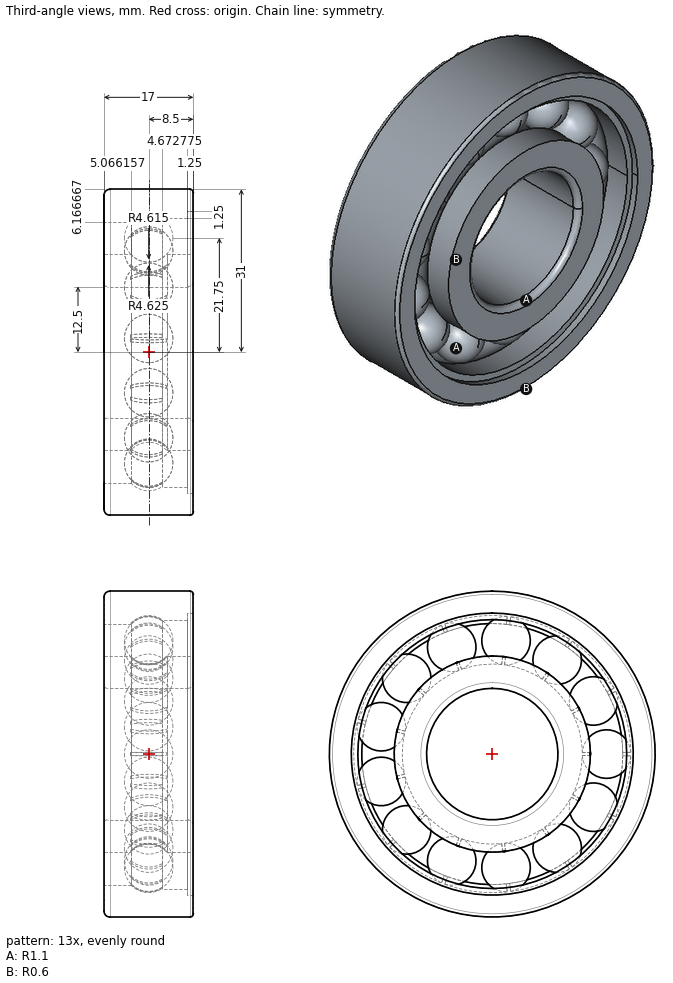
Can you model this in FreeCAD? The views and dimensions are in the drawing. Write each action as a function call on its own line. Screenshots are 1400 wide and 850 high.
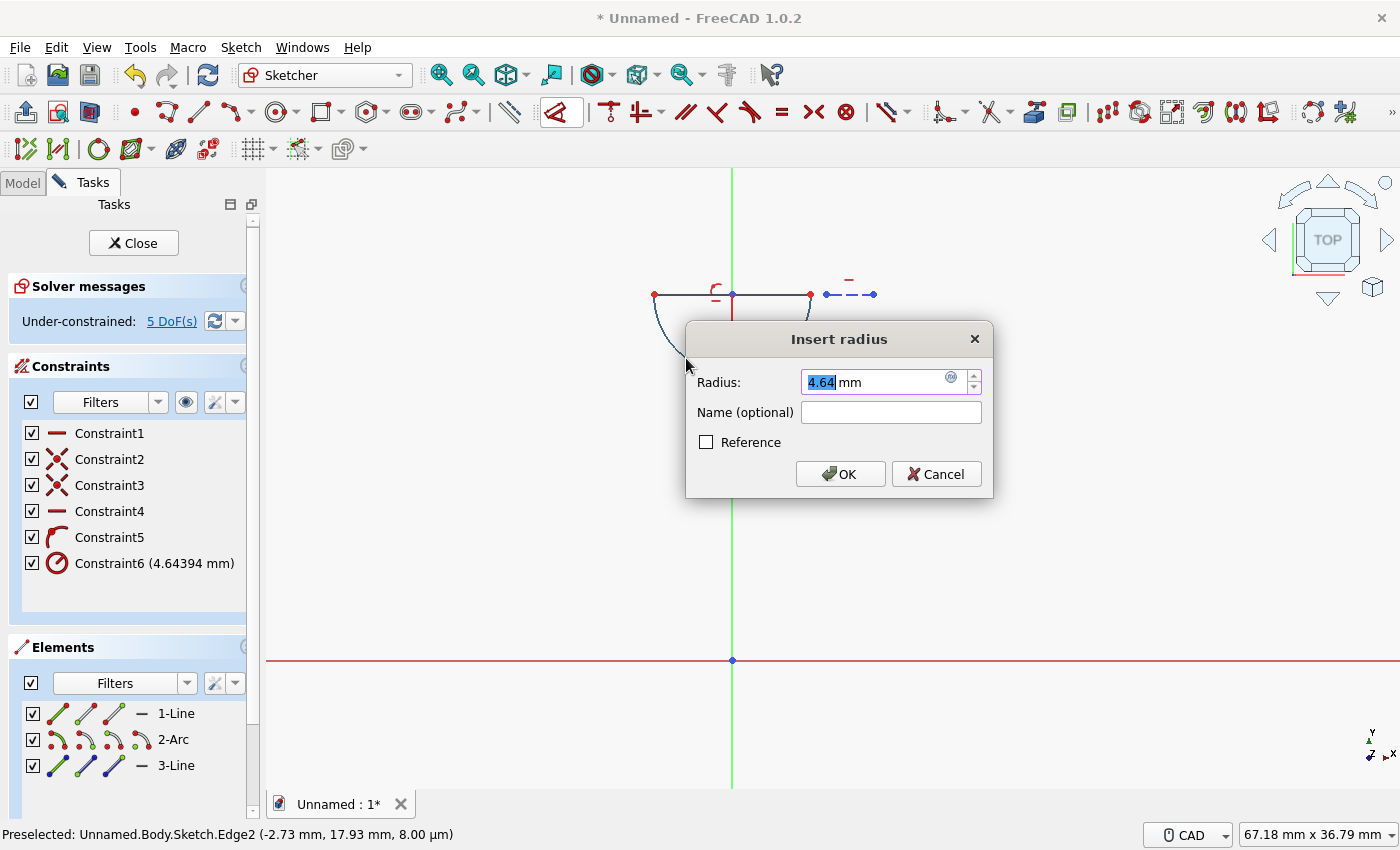
text(4.625)
key(Return)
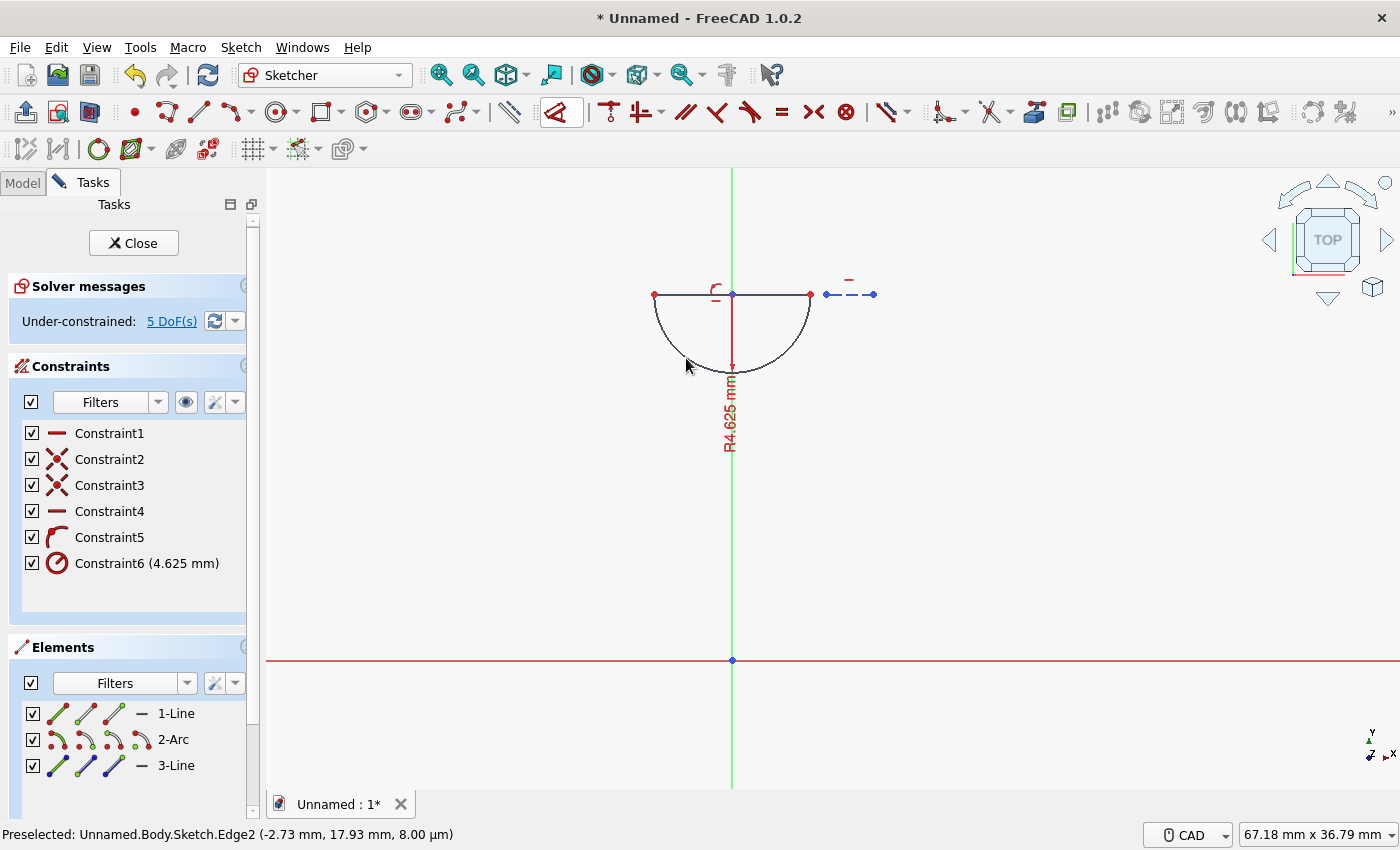
click(810, 295)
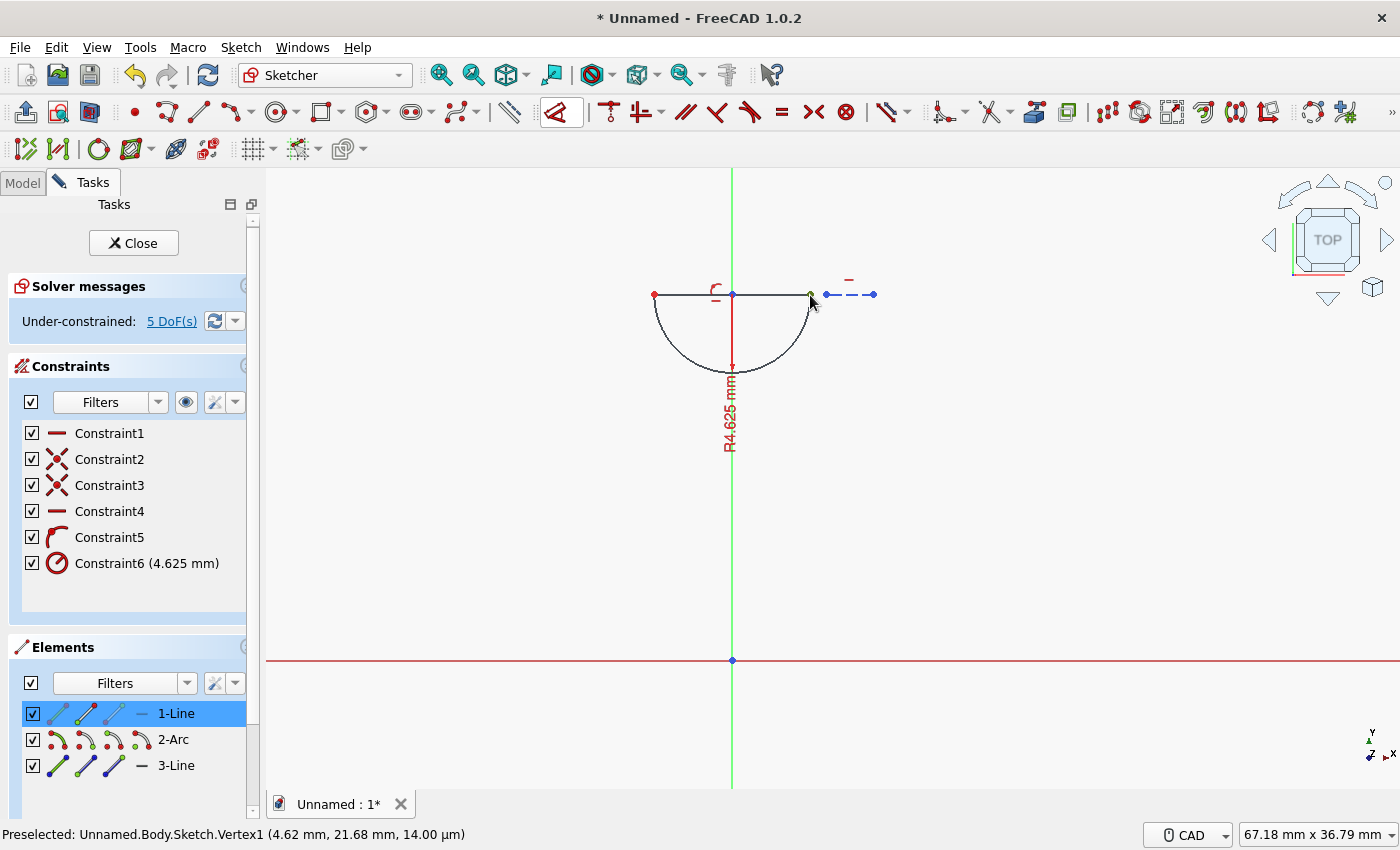
key(i)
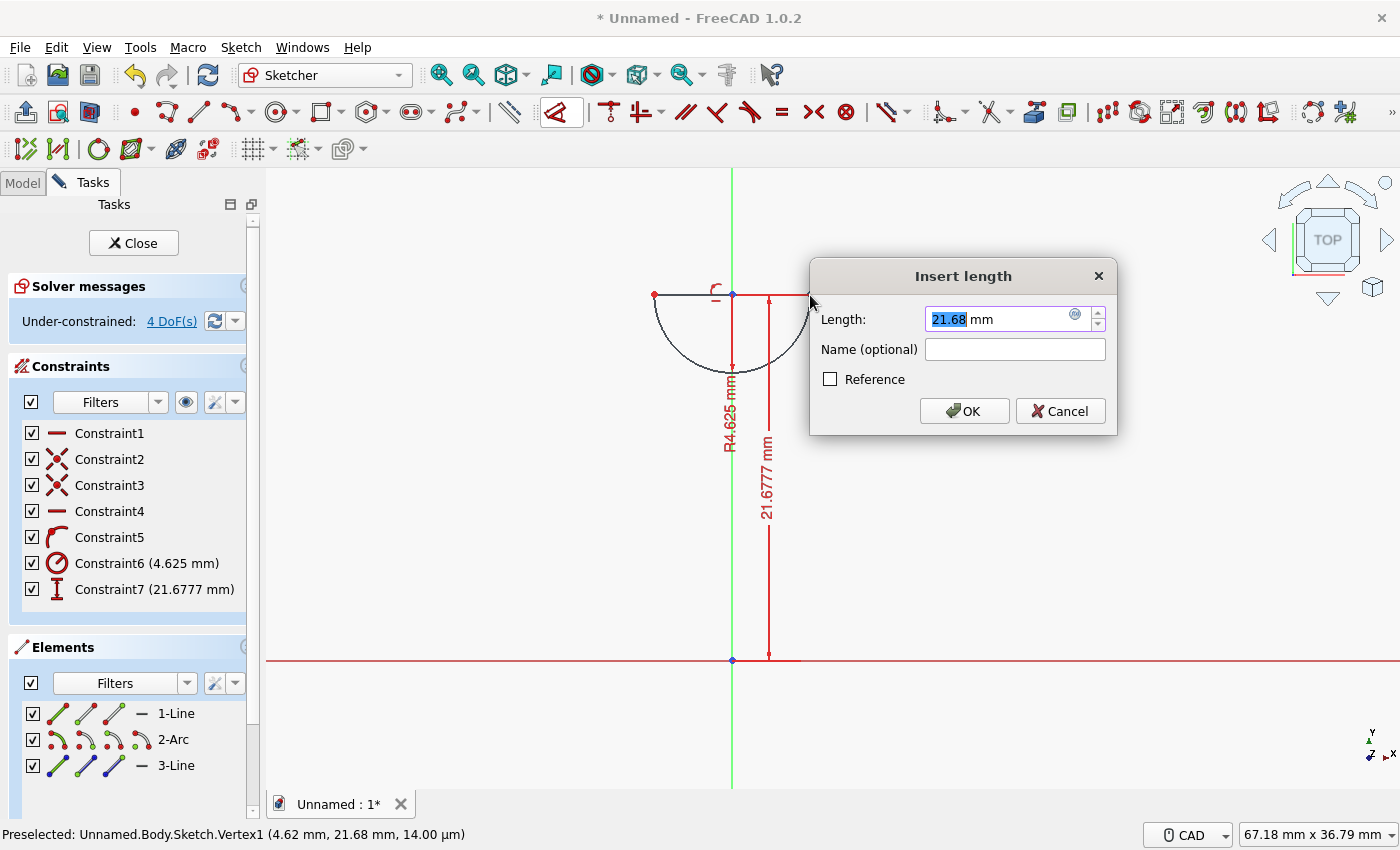
text(21.75)
key(Return)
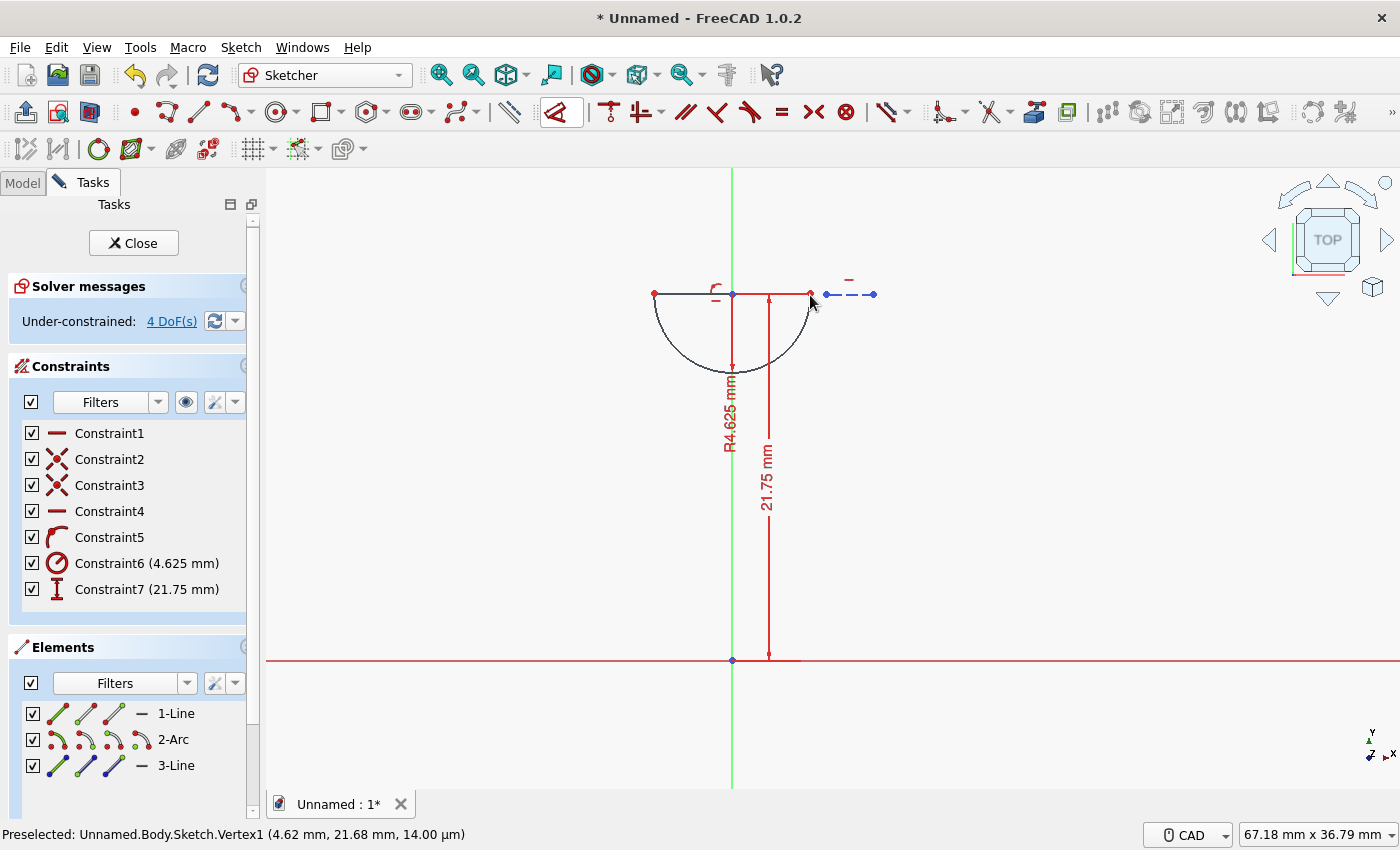
click(826, 295)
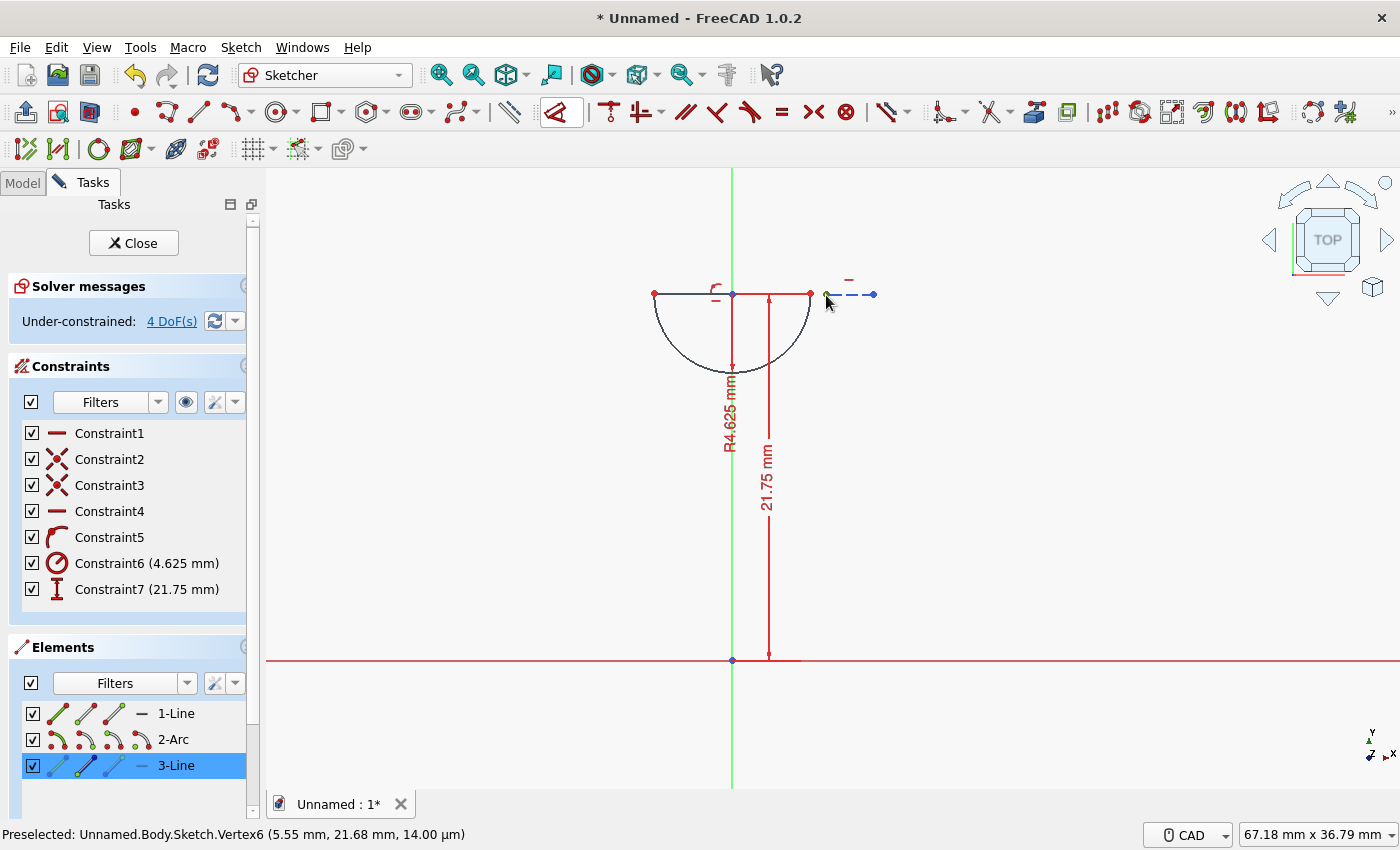
click(578, 112)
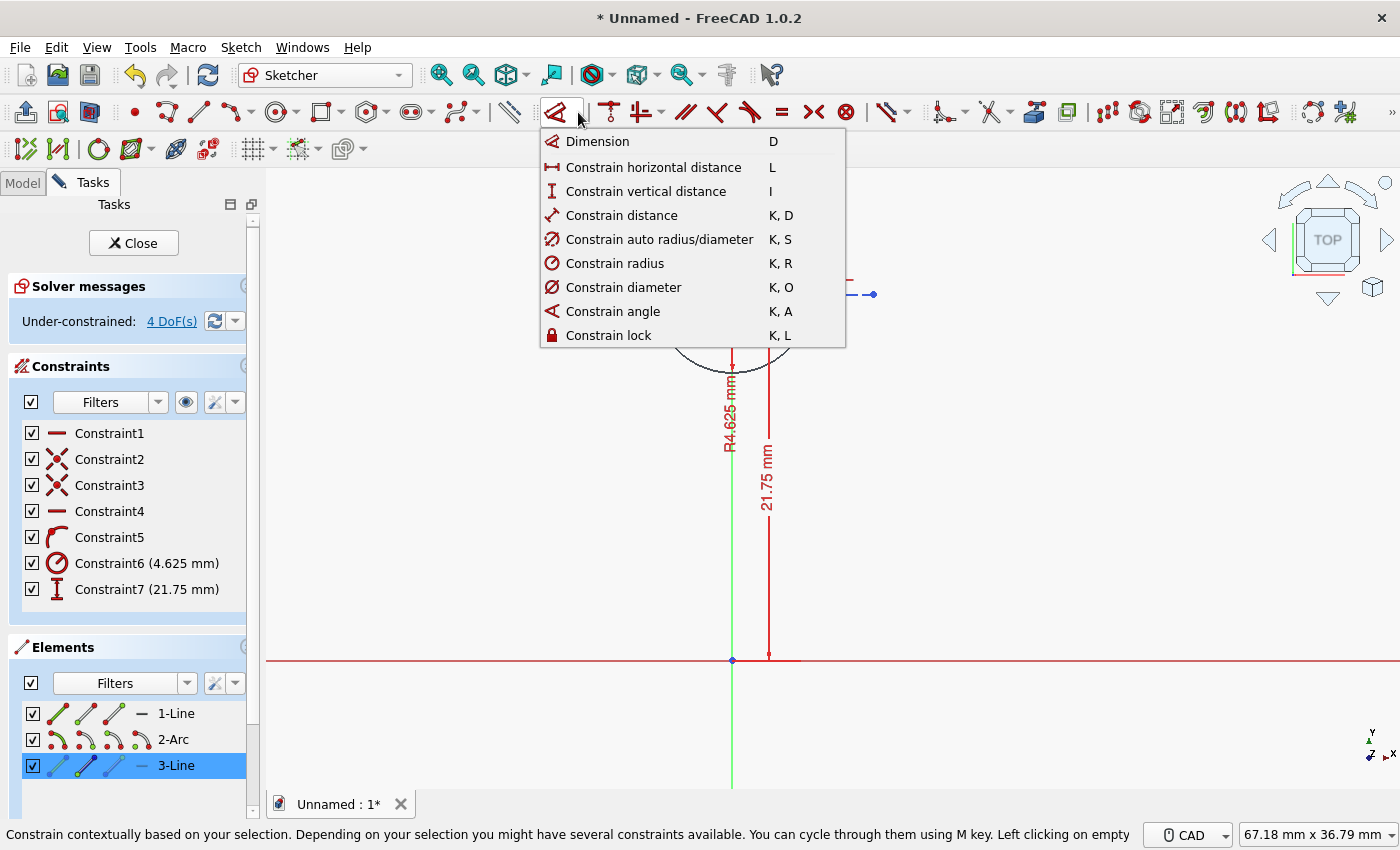
click(693, 191)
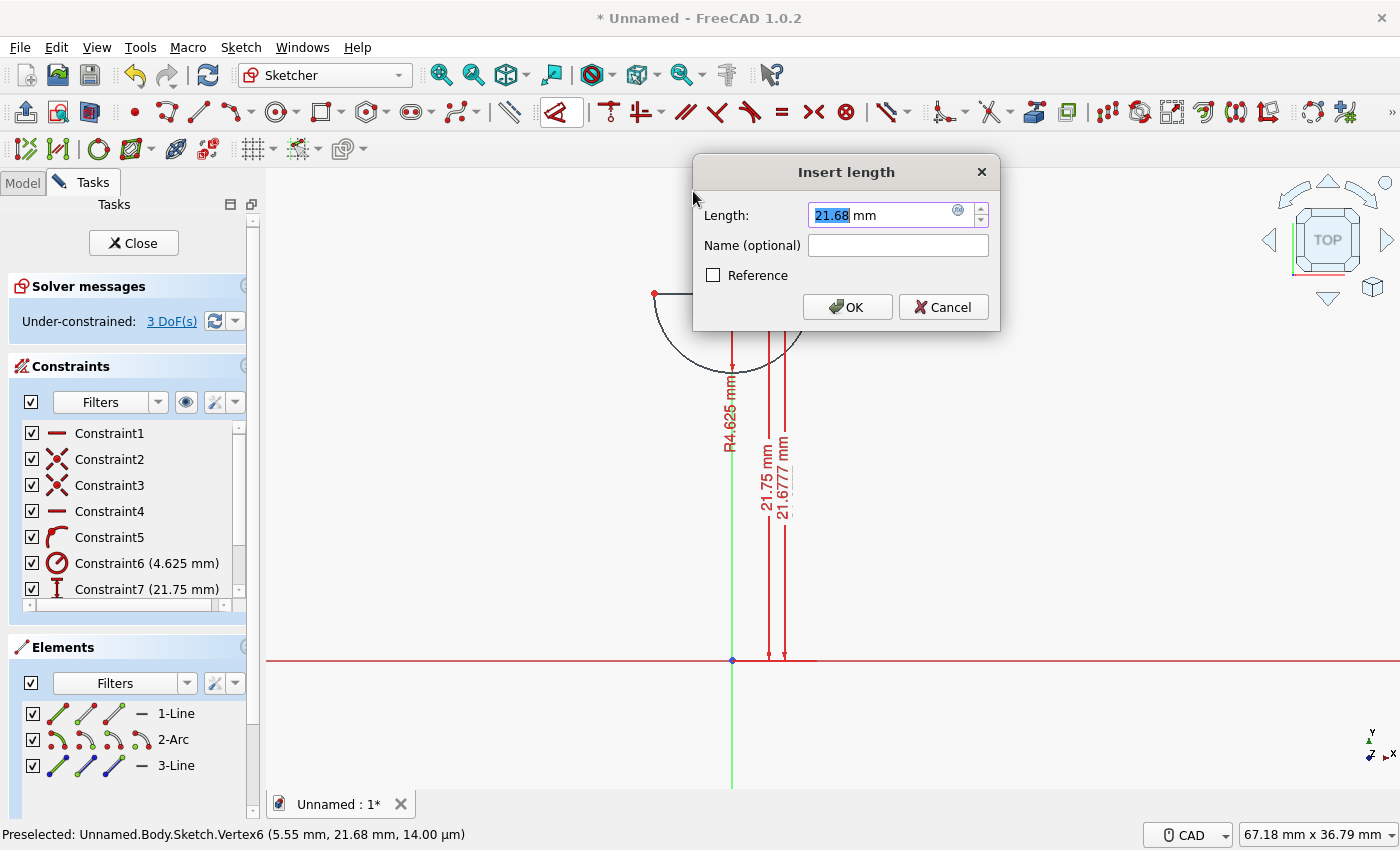
text(21.75)
key(Return)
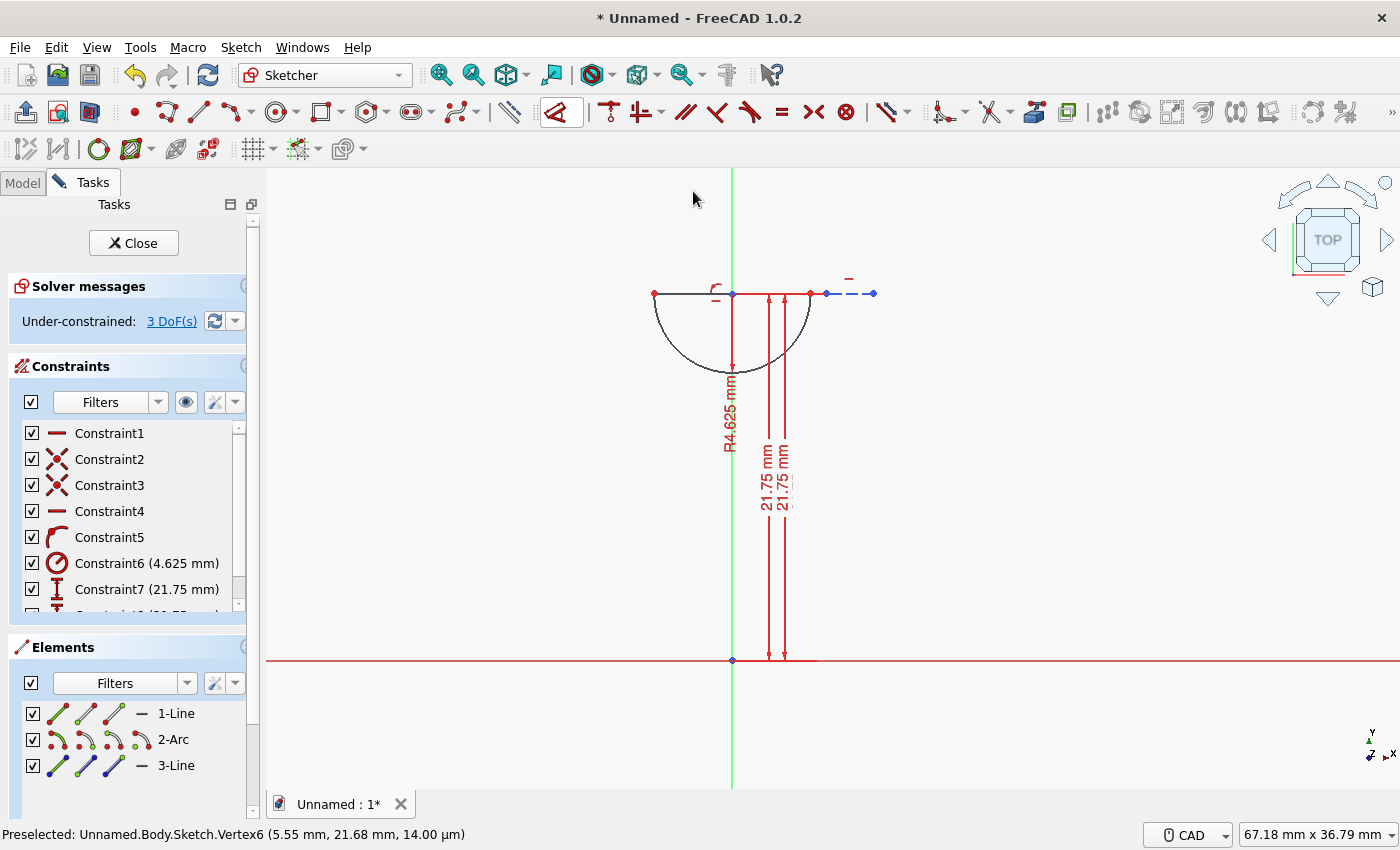
click(732, 295)